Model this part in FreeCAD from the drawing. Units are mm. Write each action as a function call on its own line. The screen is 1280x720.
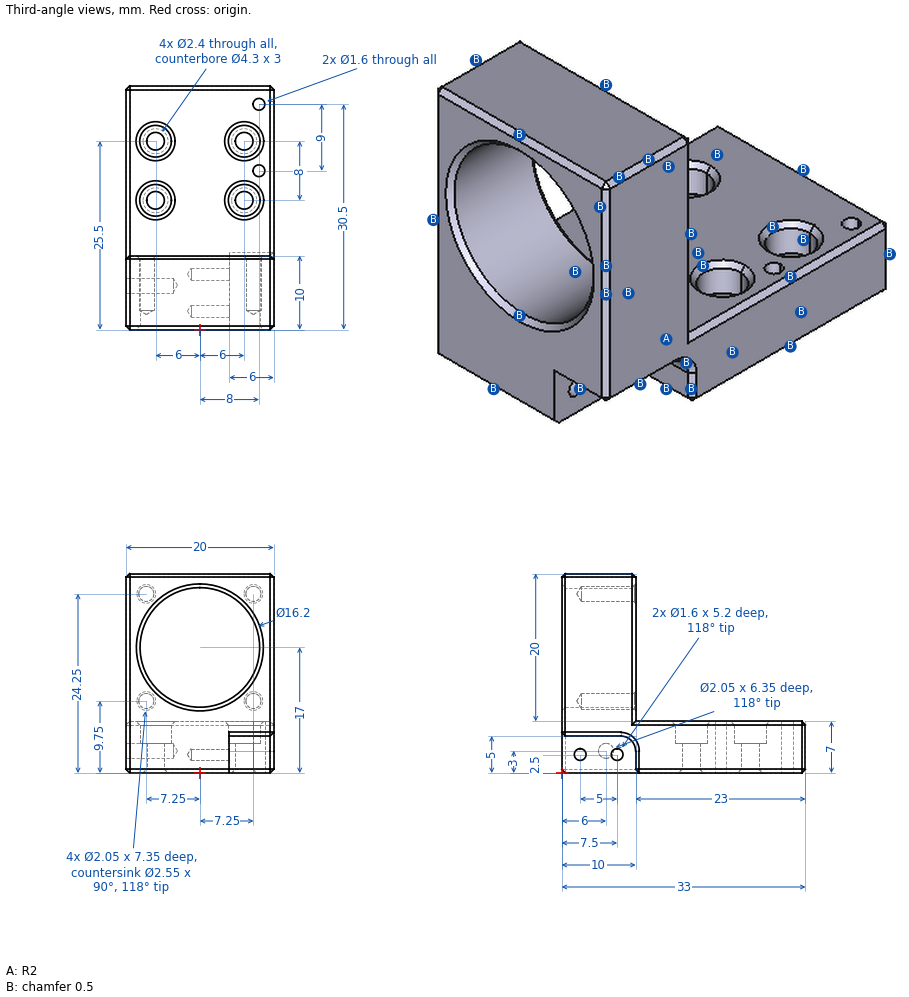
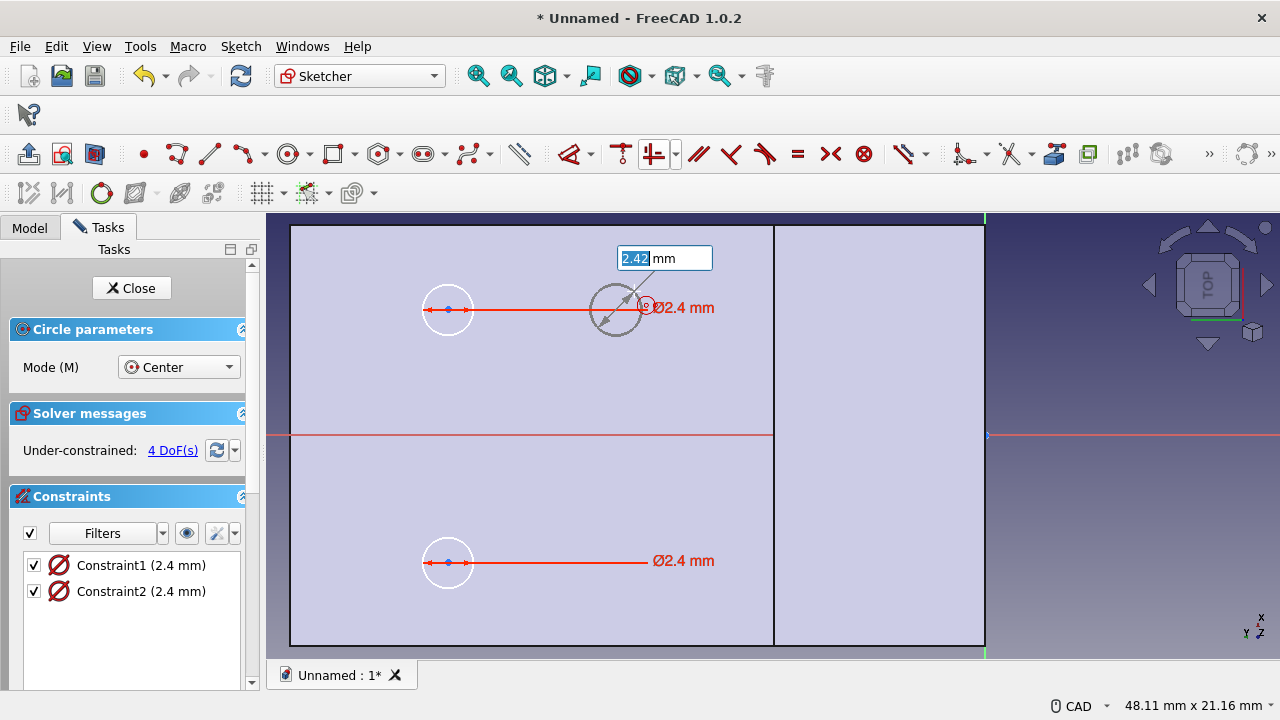
text(2.4)
key(Return)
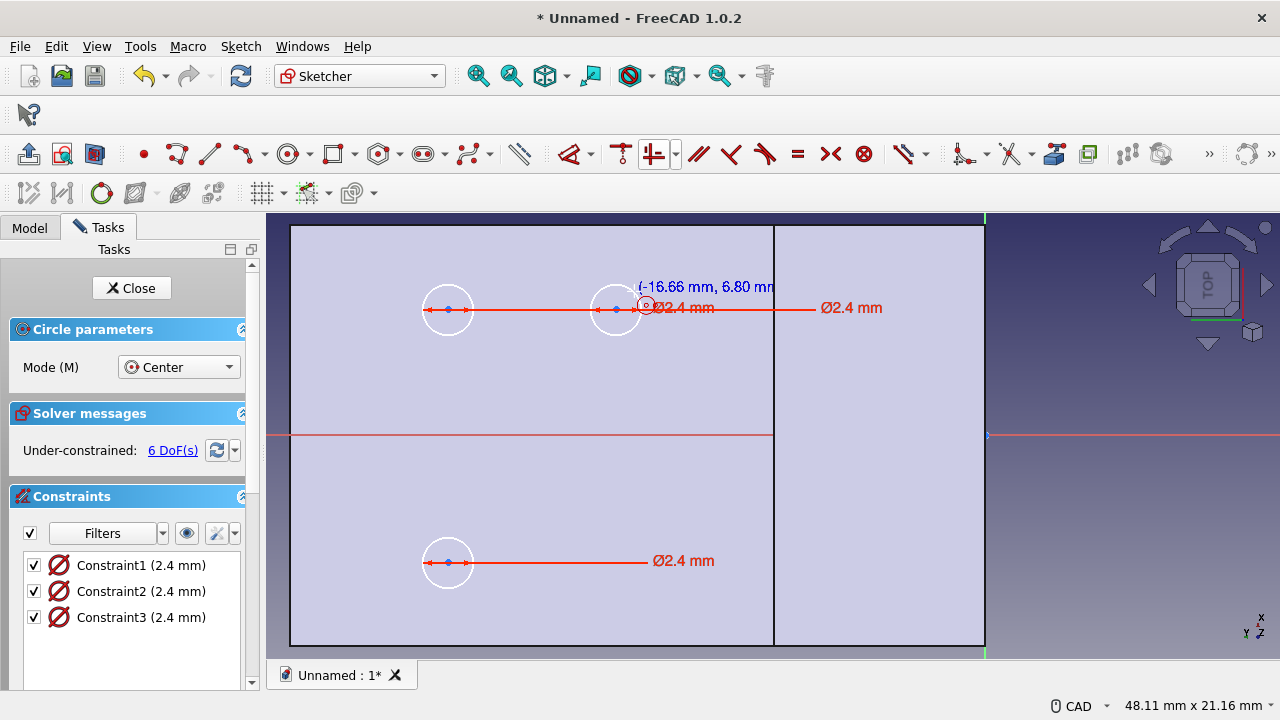
click(616, 562)
move(634, 544)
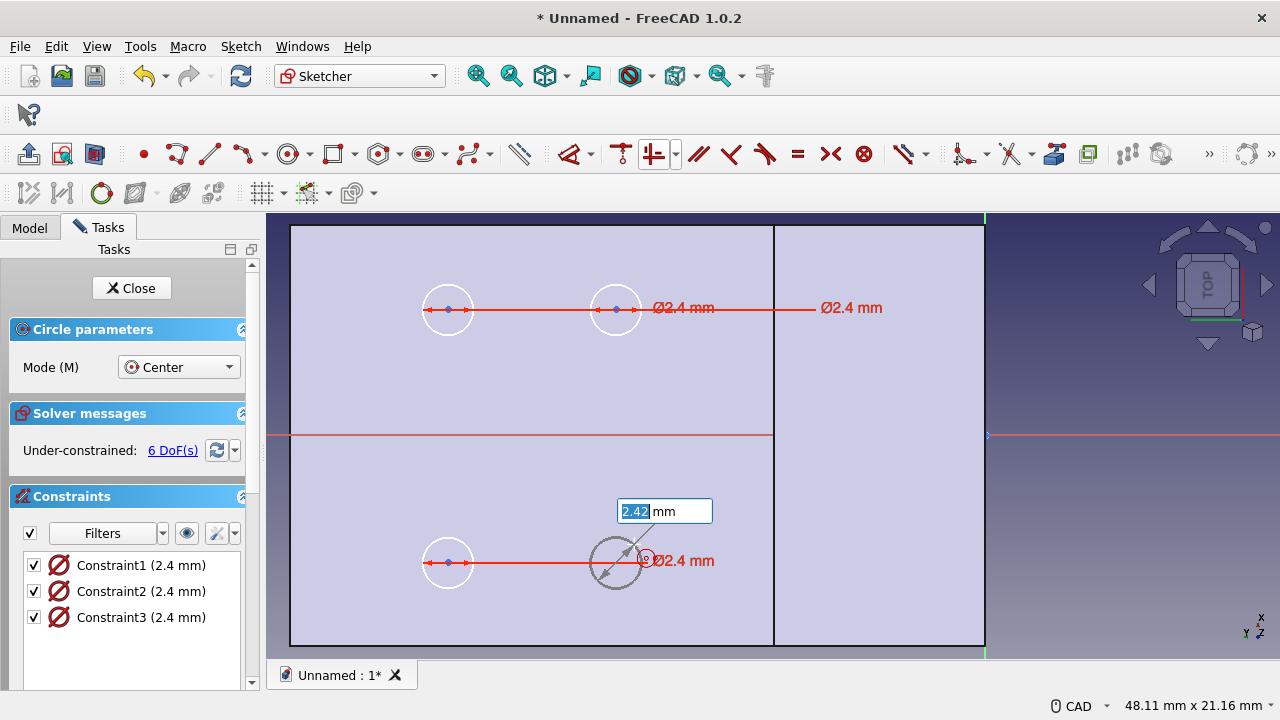
text(2.4)
key(Return)
key(Escape)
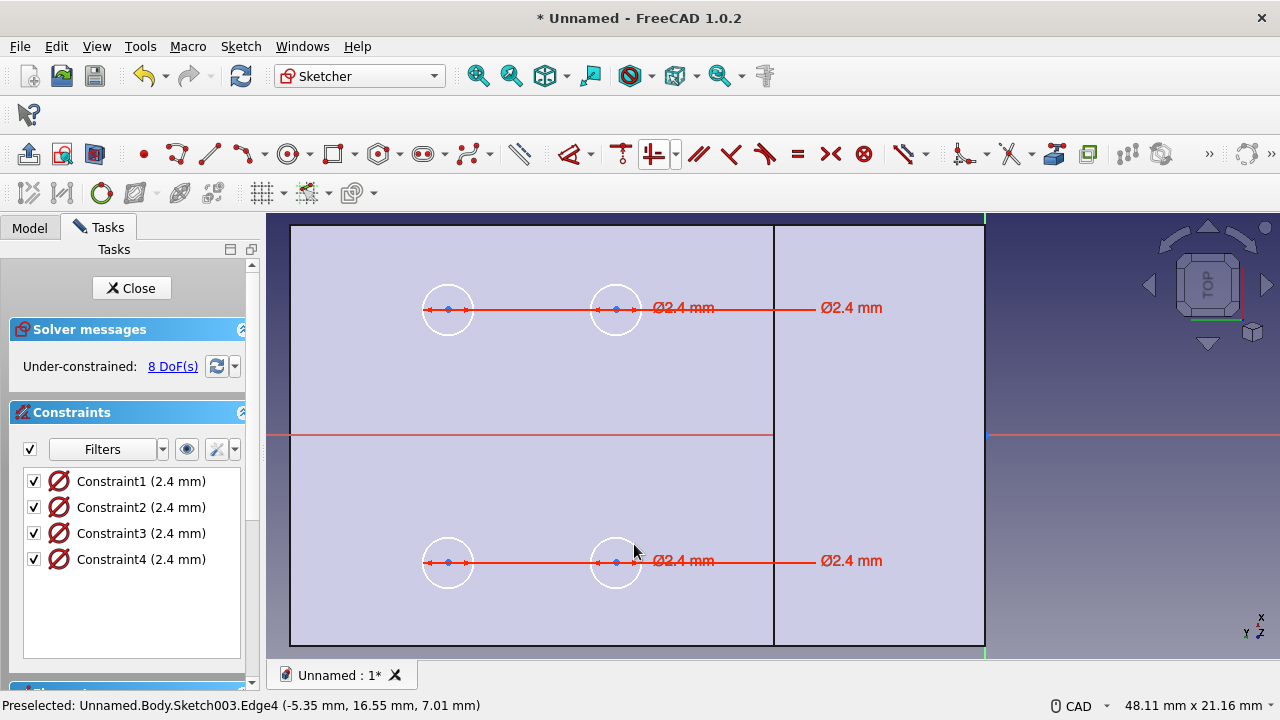
click(448, 563)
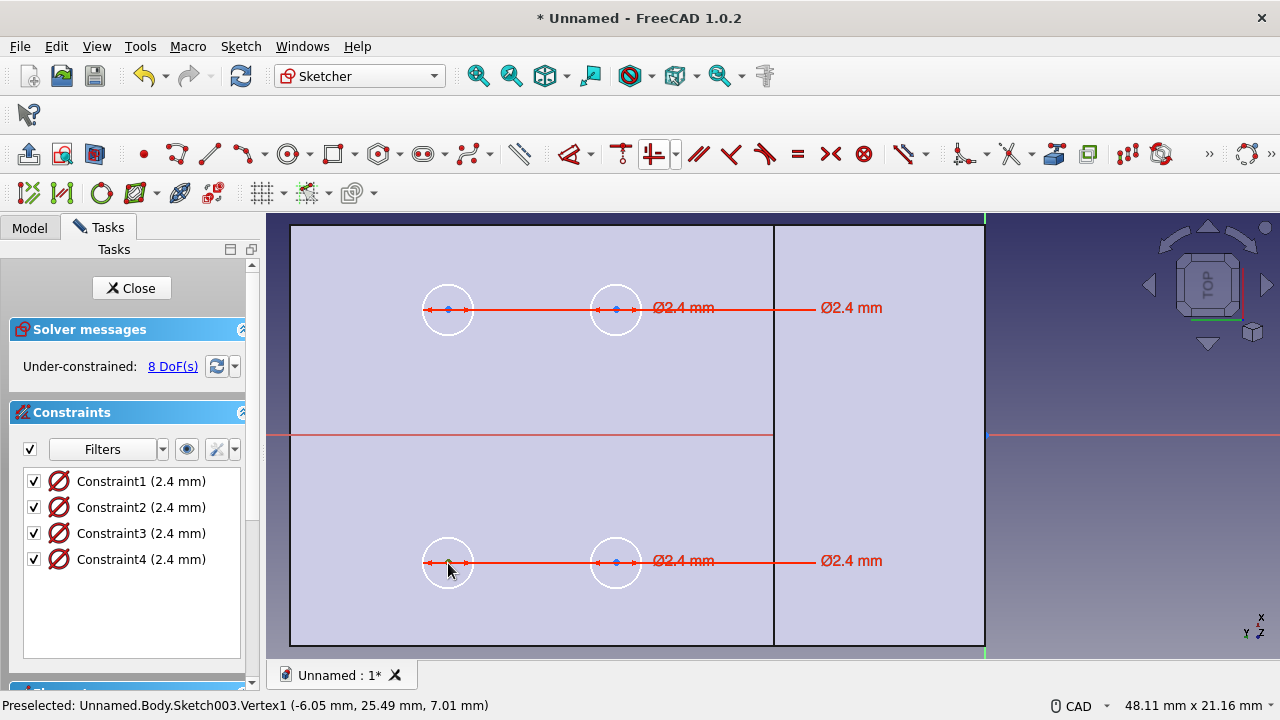
click(448, 310)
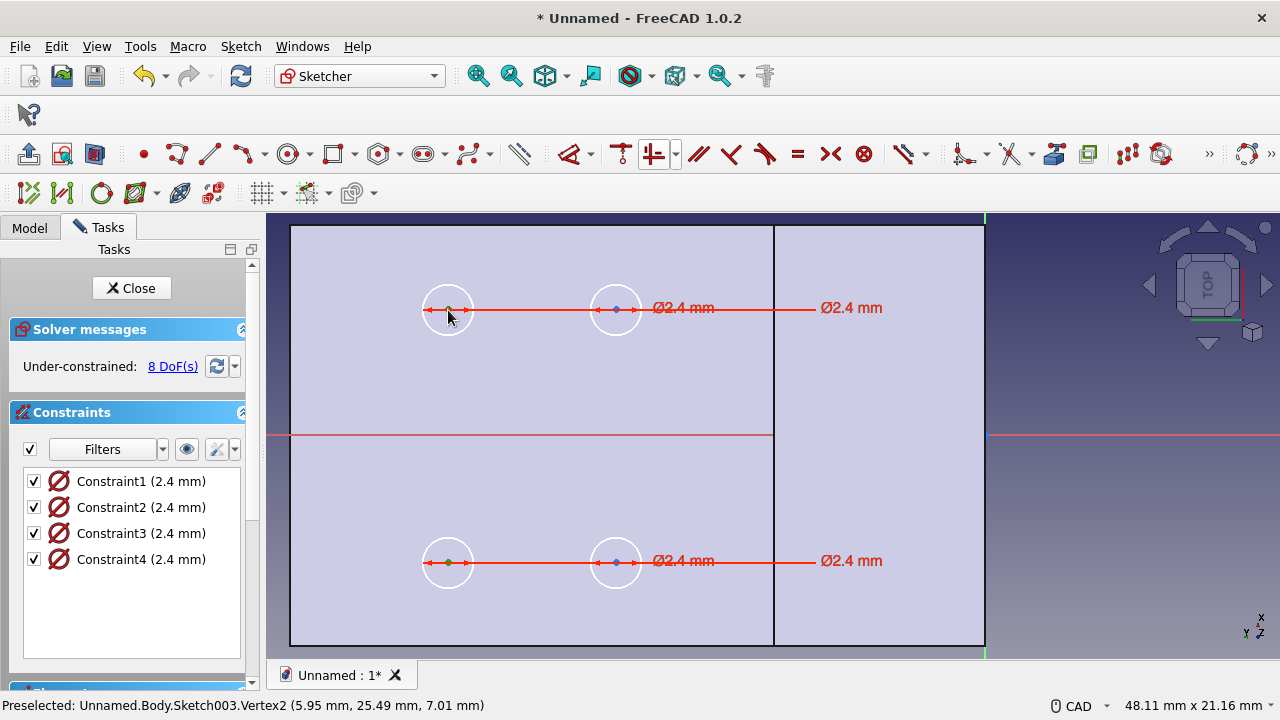
key(v)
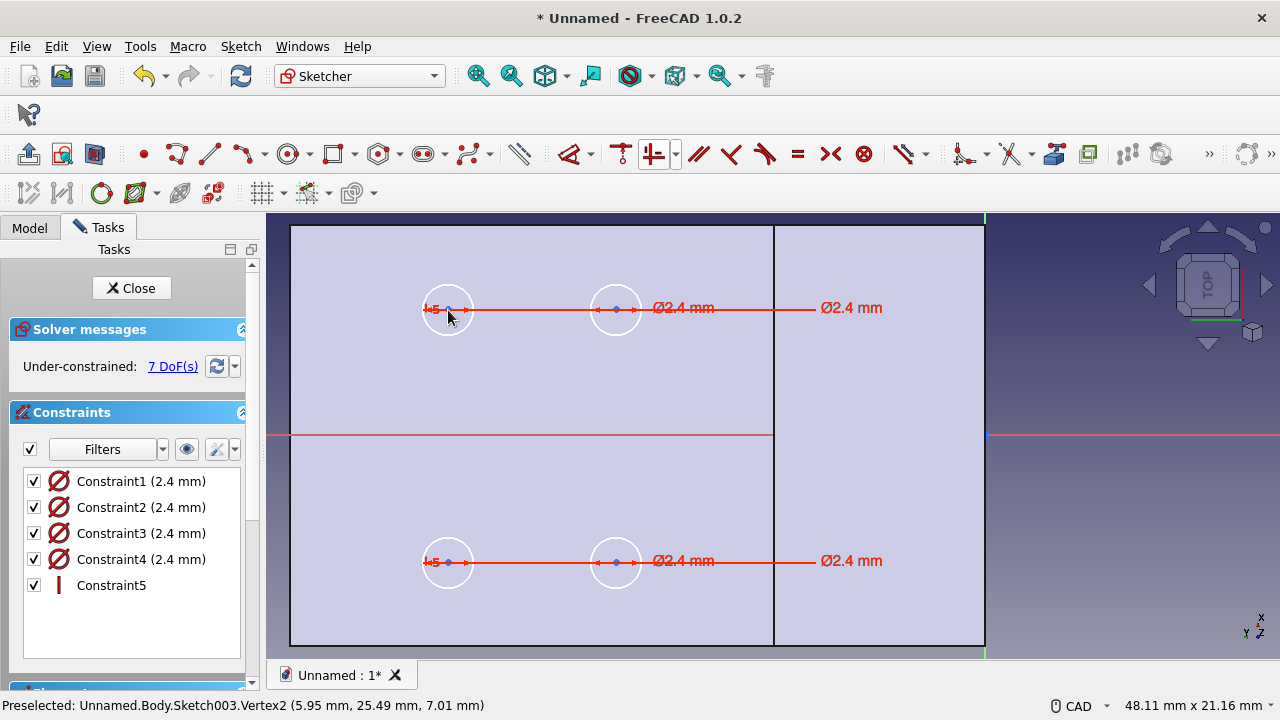
click(448, 310)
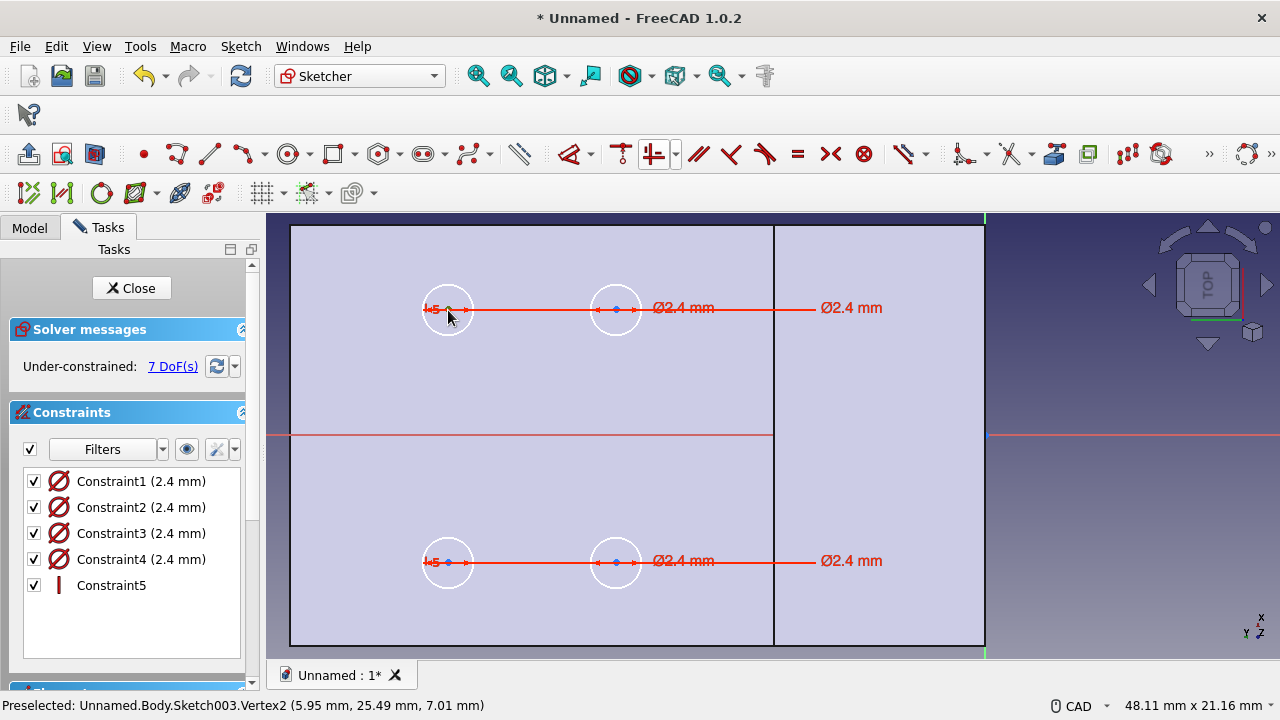
click(616, 310)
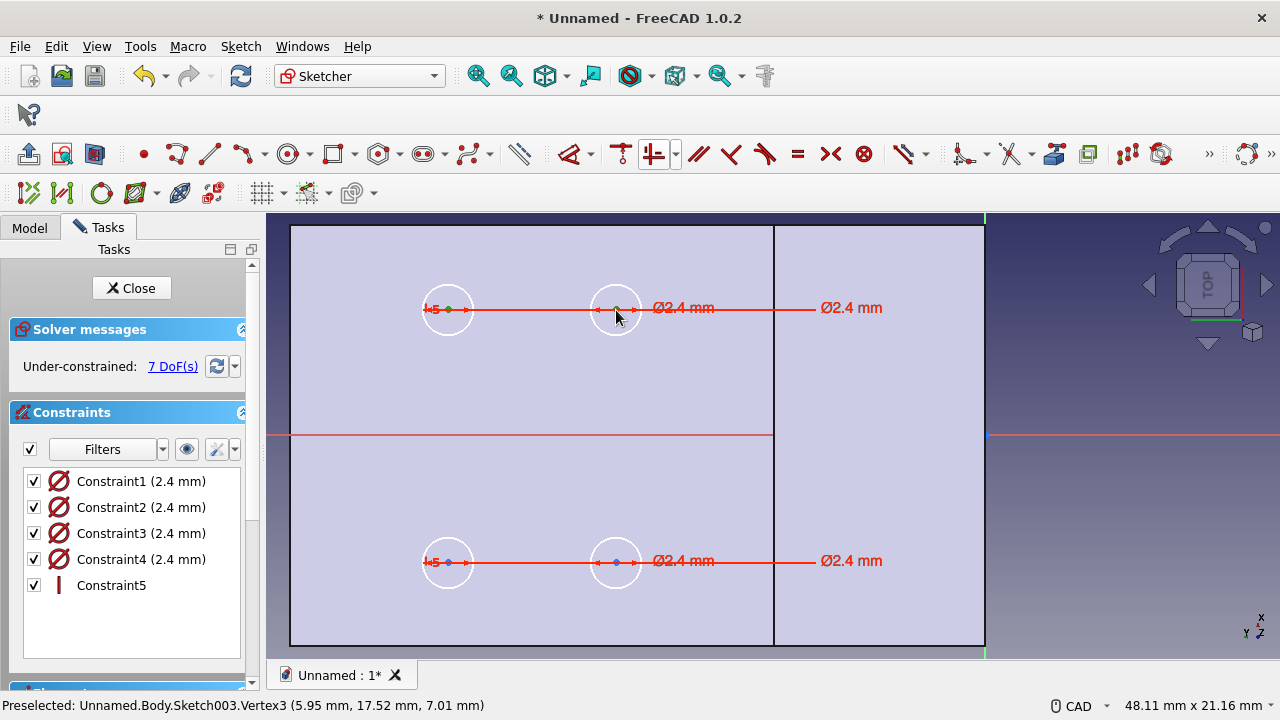
key(h)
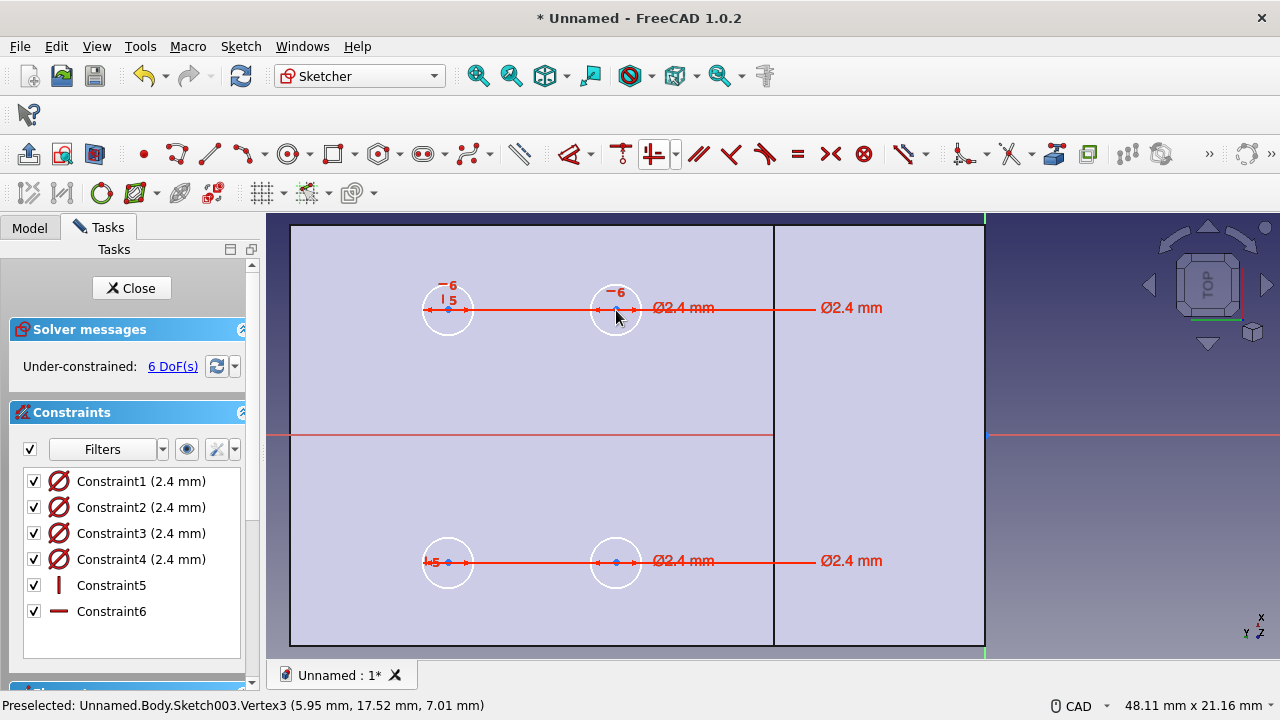
click(616, 310)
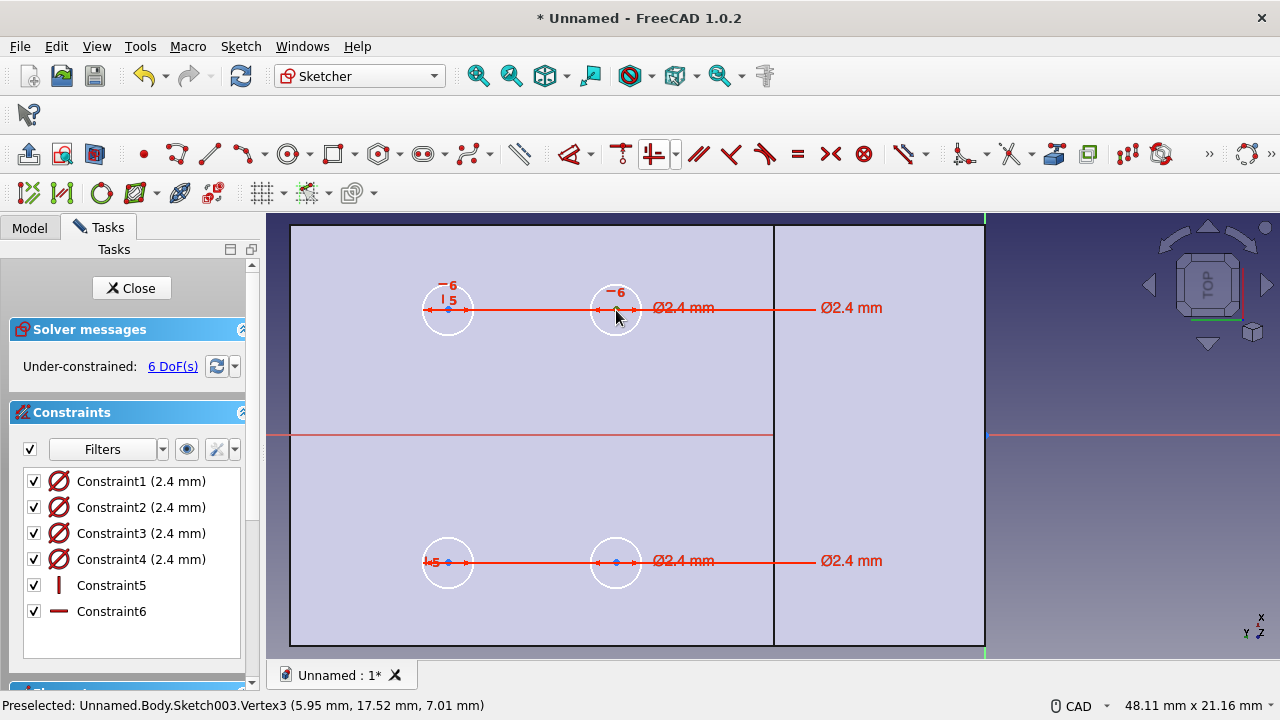
click(616, 563)